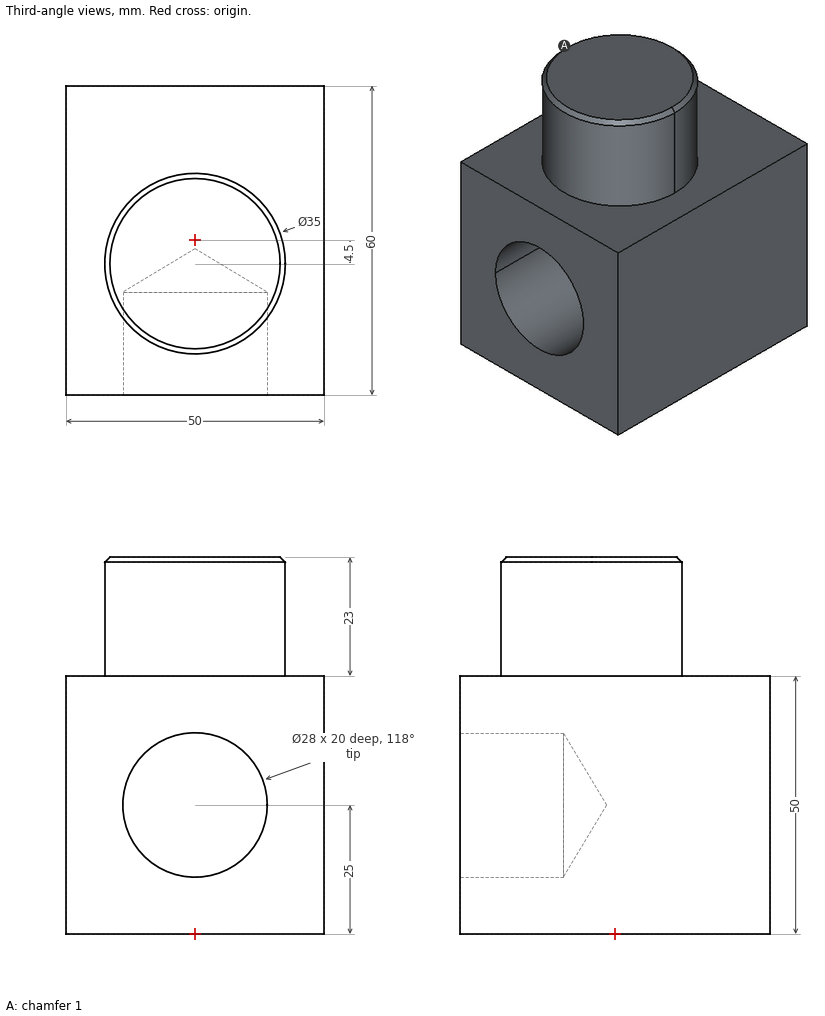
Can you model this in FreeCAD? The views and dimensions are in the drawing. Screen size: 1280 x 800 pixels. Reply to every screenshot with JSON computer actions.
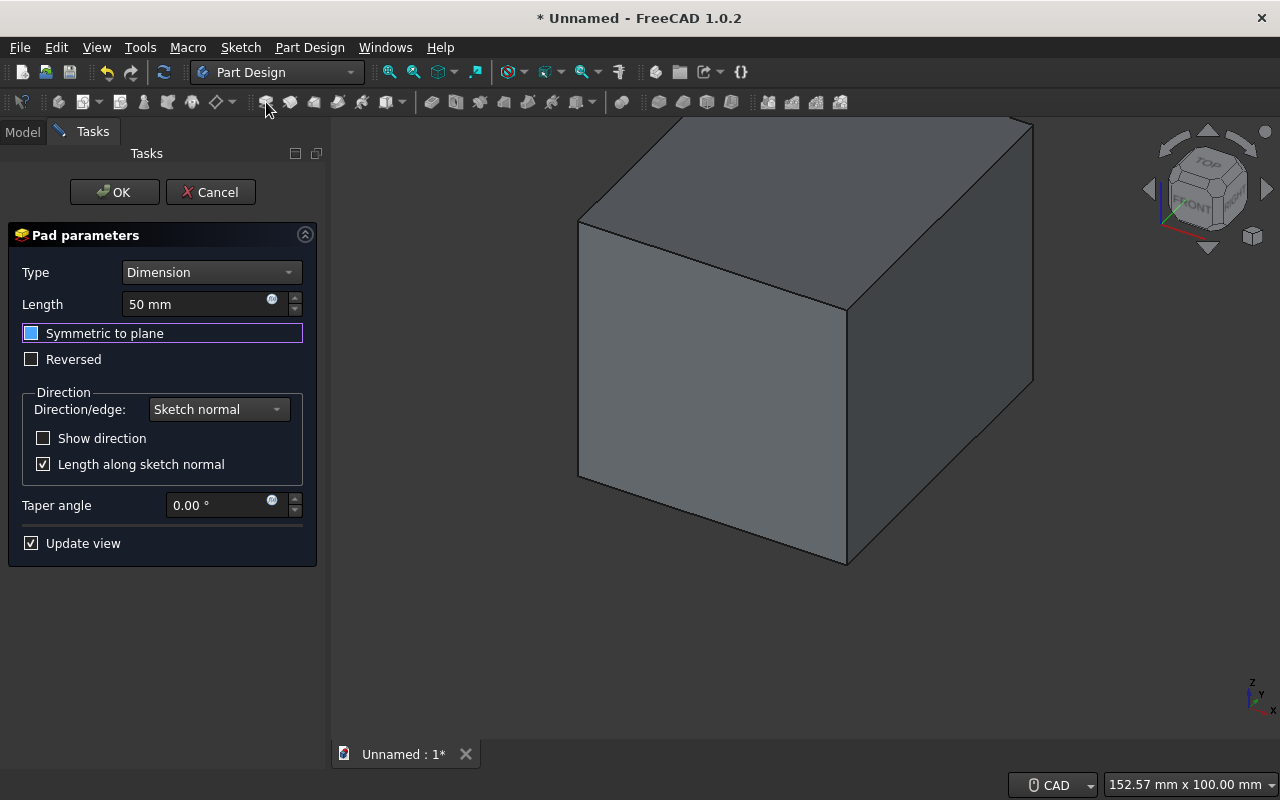
{"action": "left_click", "coordinate": [115, 192]}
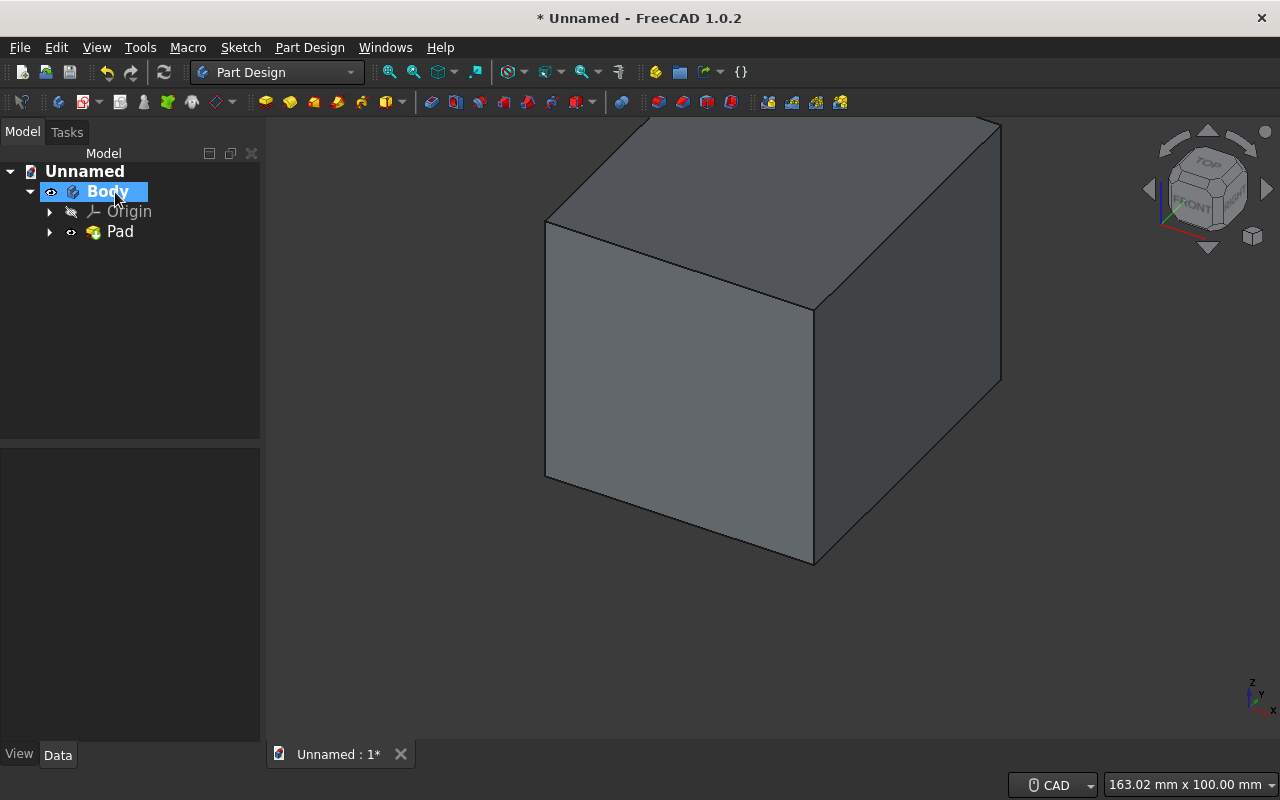
{"action": "left_click", "coordinate": [390, 72]}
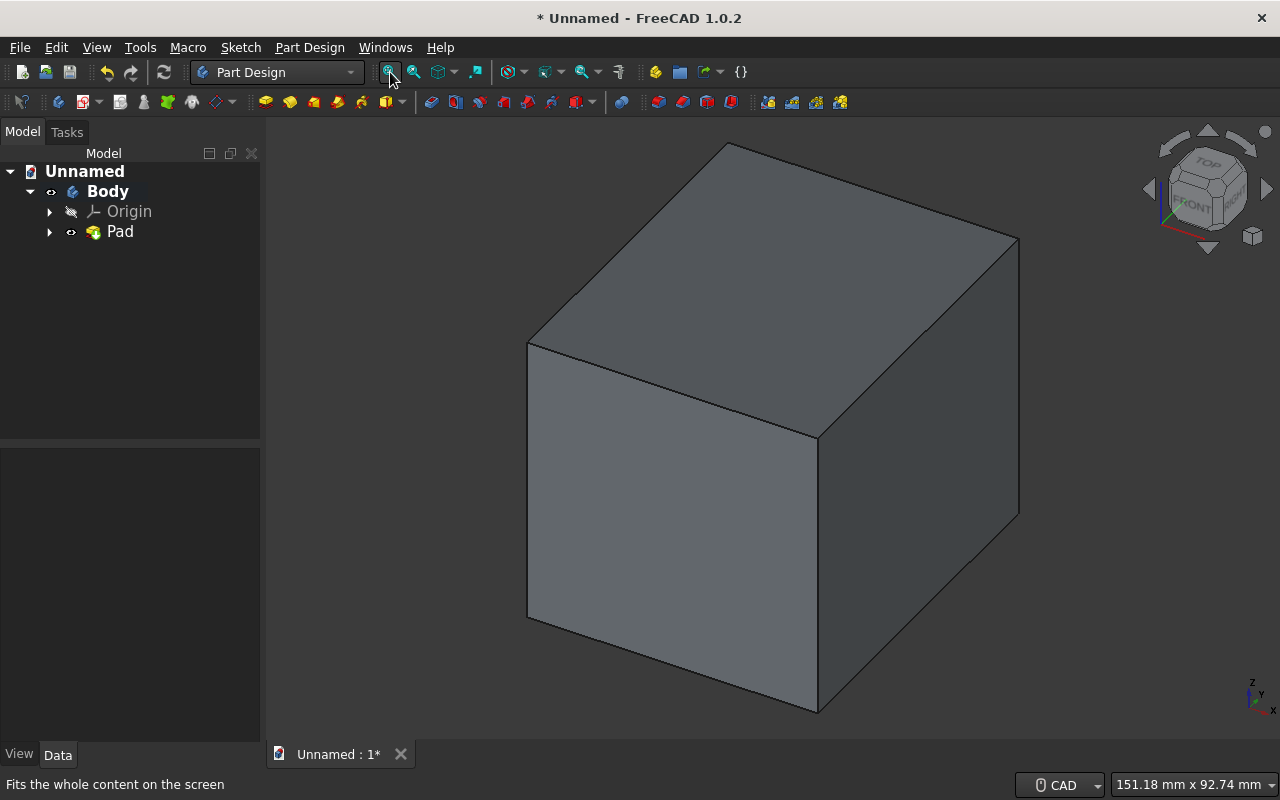
{"action": "left_click", "coordinate": [773, 290]}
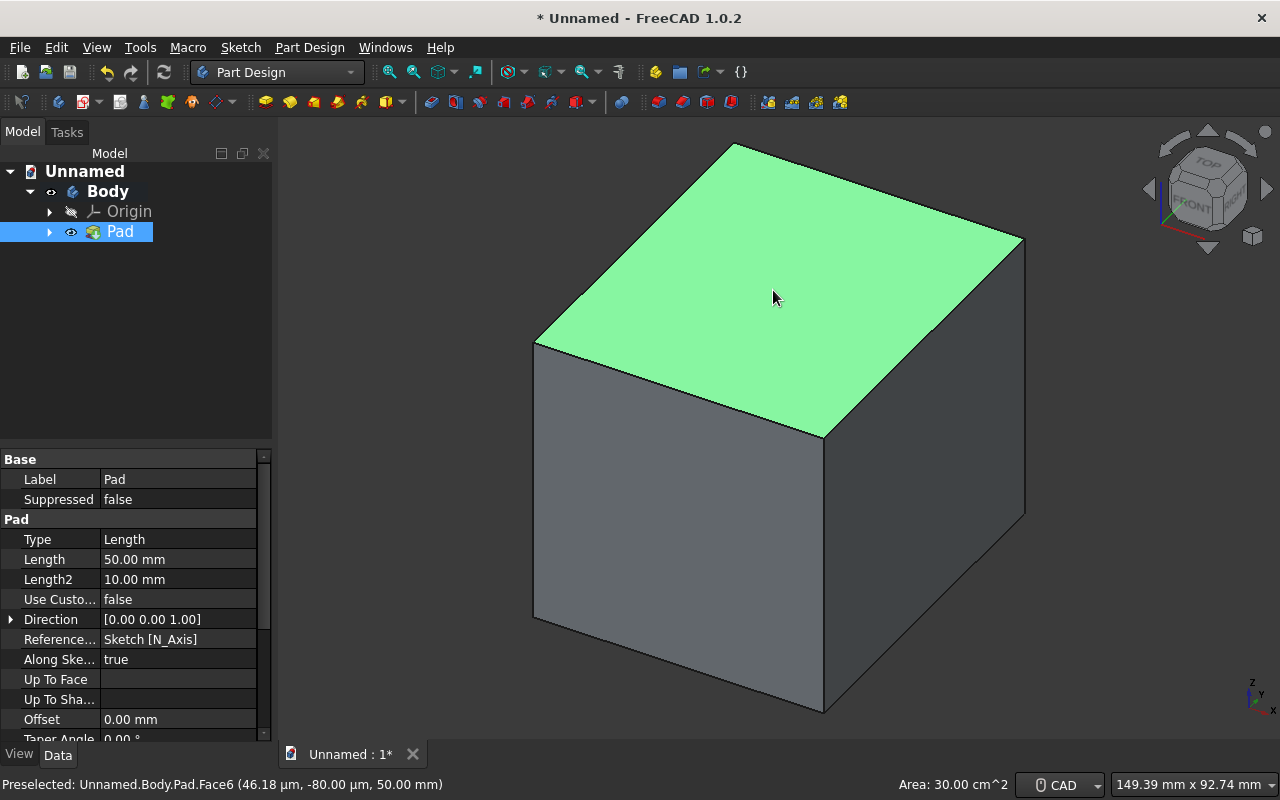
{"action": "left_click", "coordinate": [84, 102]}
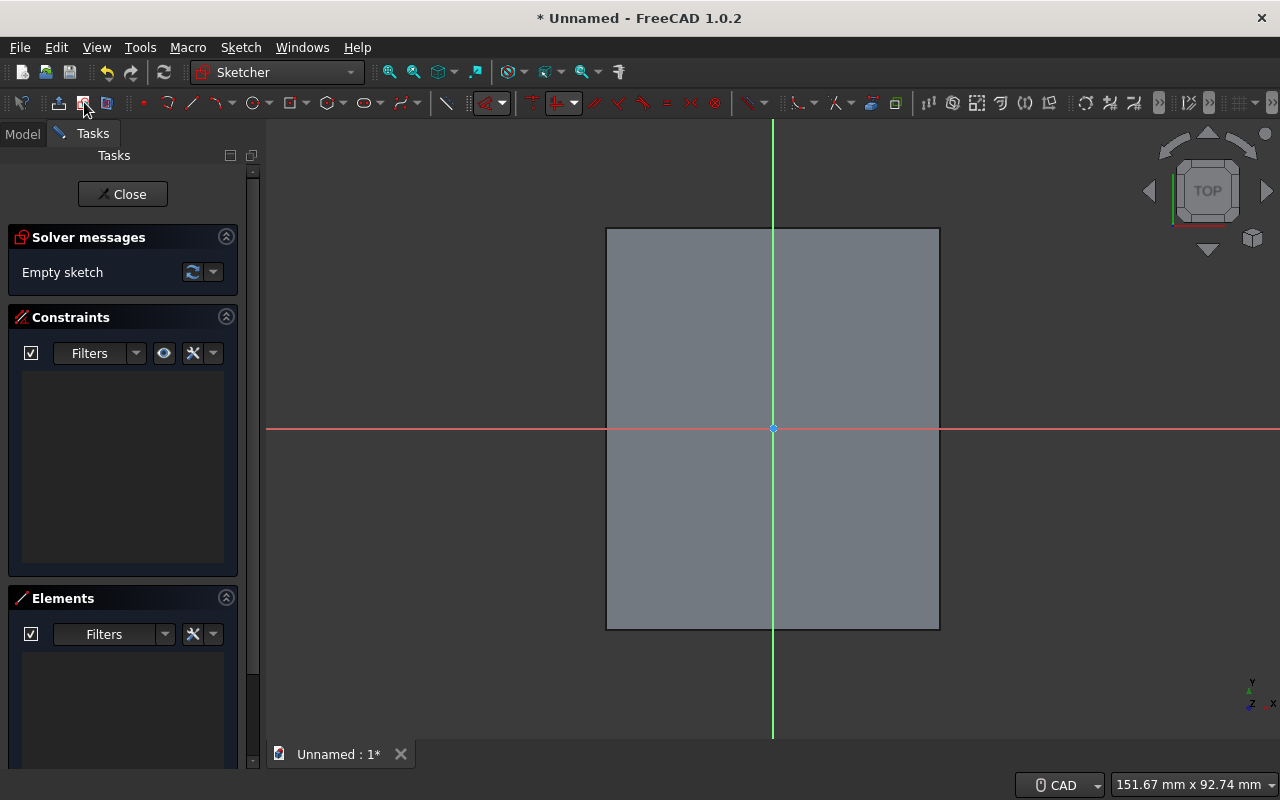
{"action": "scroll", "coordinate": [856, 496], "scroll_direction": "up", "scroll_amount": 3}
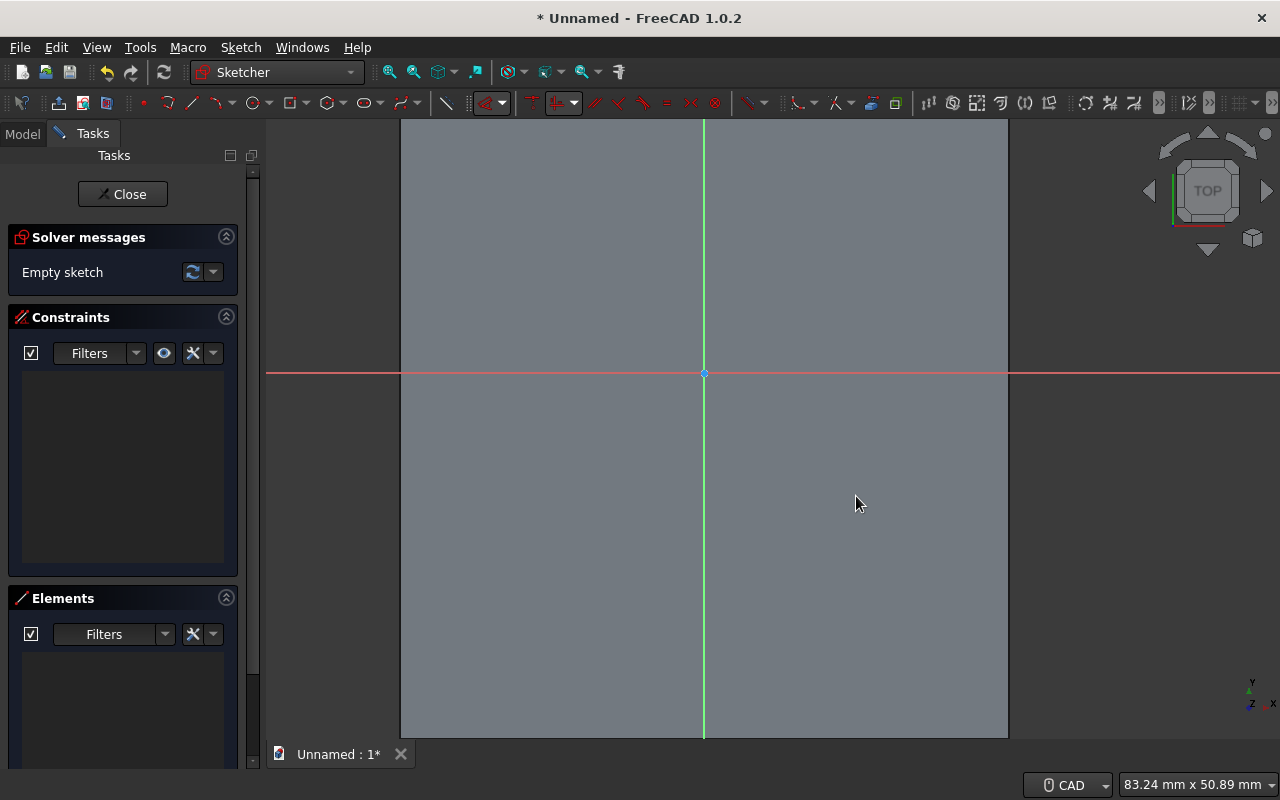
{"action": "left_click", "coordinate": [254, 104]}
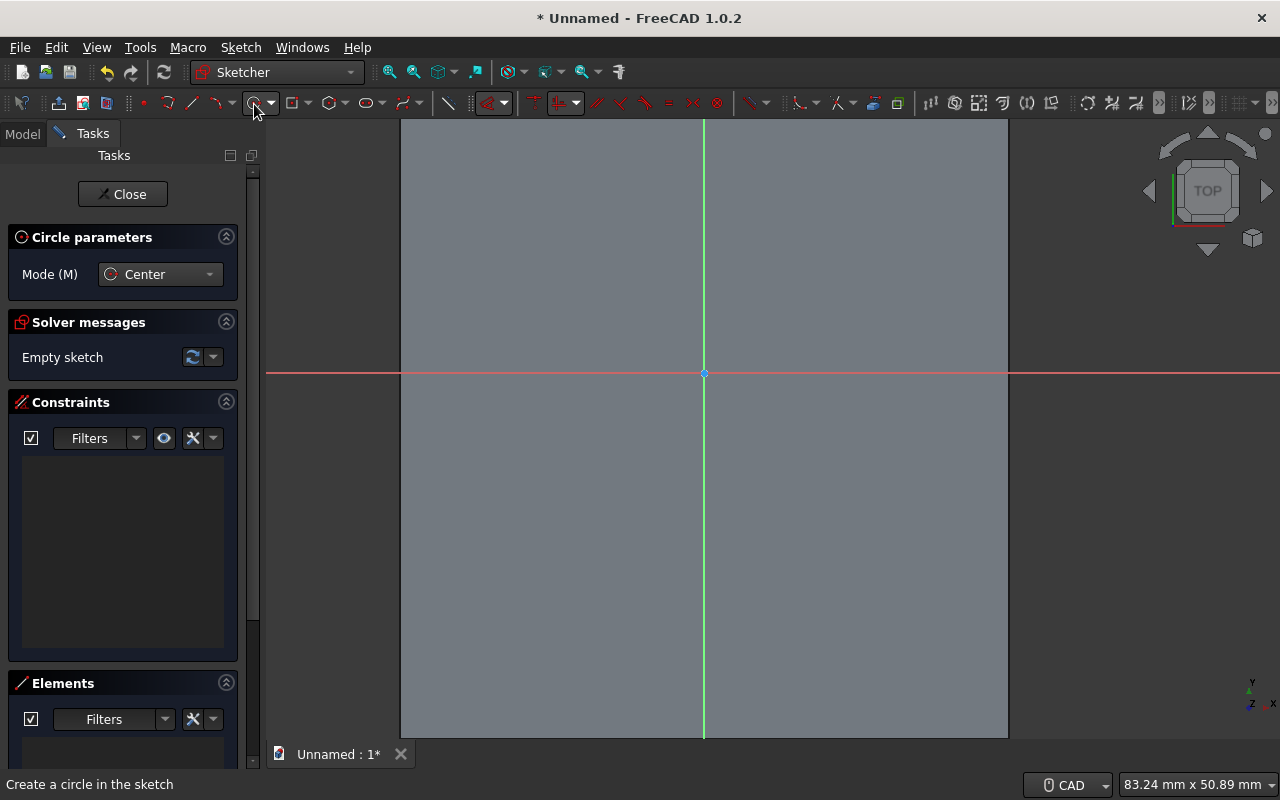
{"action": "left_click", "coordinate": [704, 428]}
{"action": "mouse_move", "coordinate": [855, 277]}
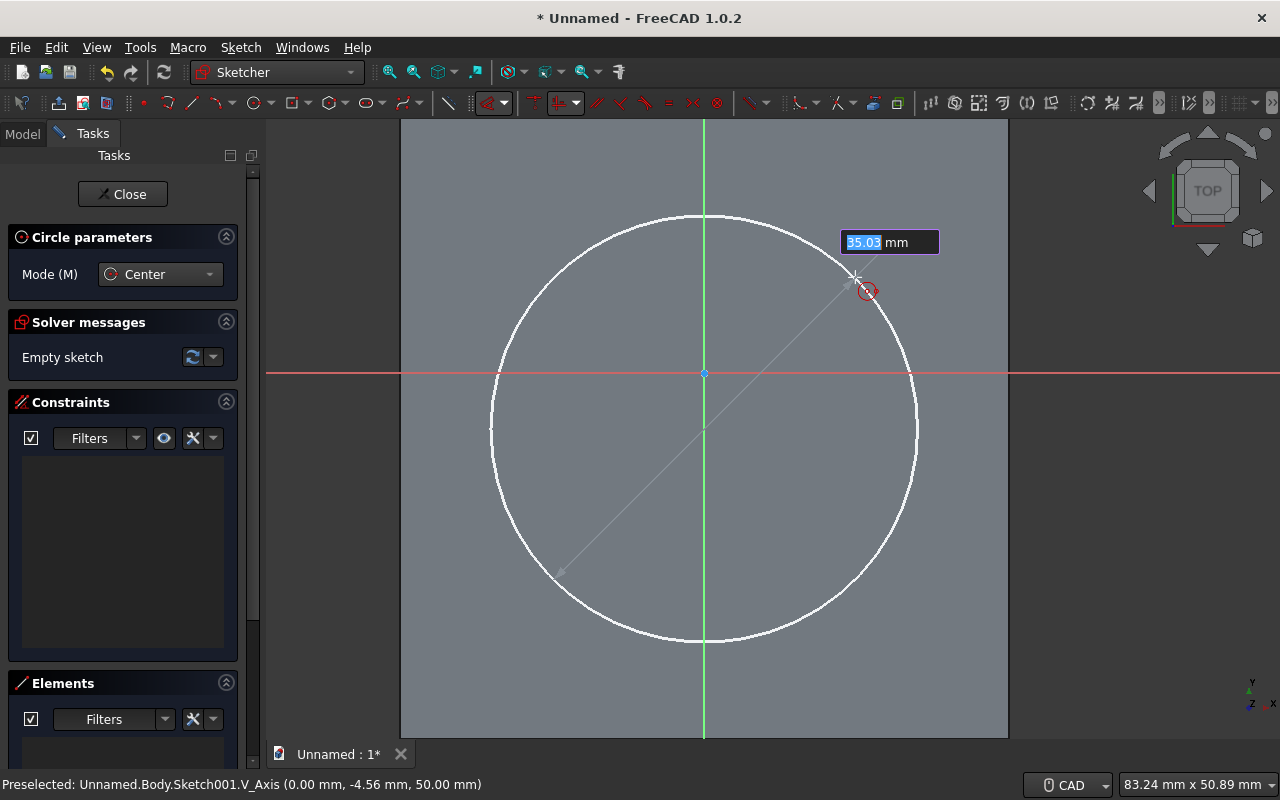
{"action": "type", "text": "35"}
{"action": "key", "text": "Return"}
{"action": "key", "text": "Escape"}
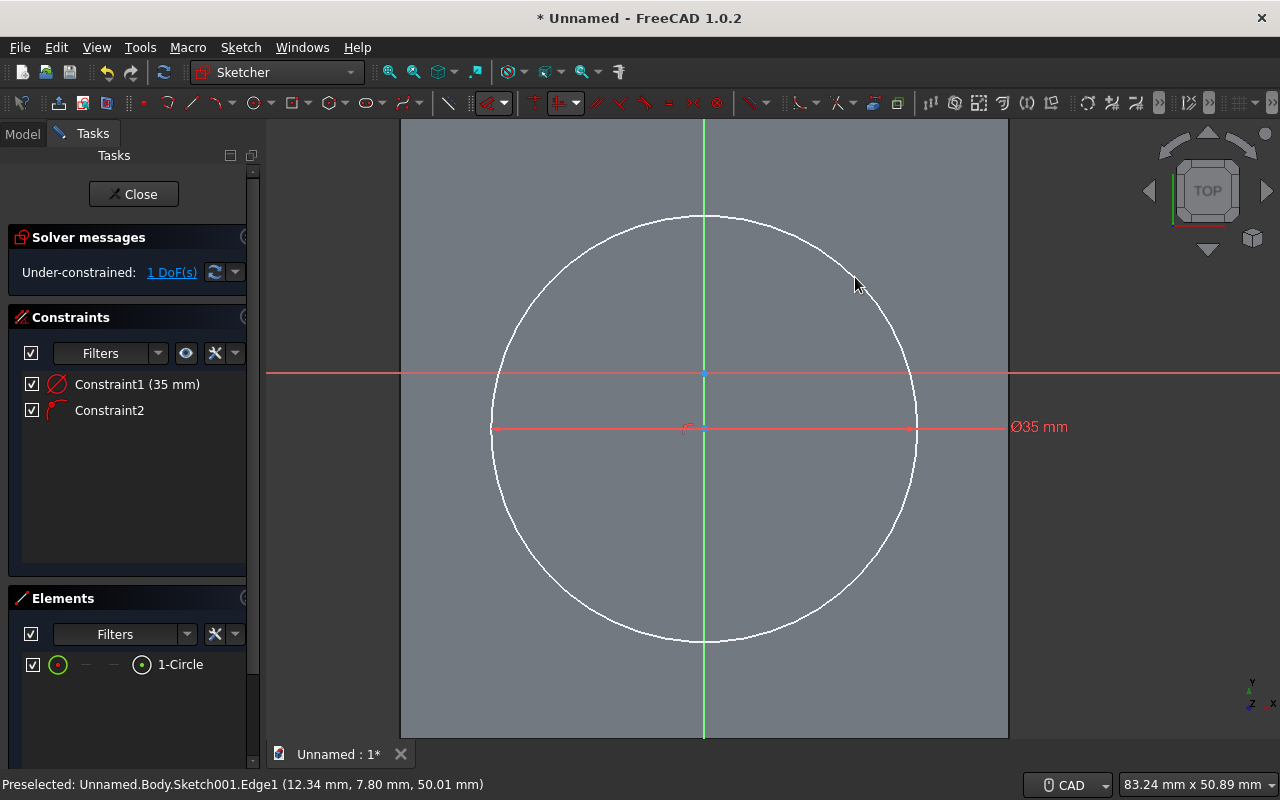
{"action": "left_click", "coordinate": [488, 104]}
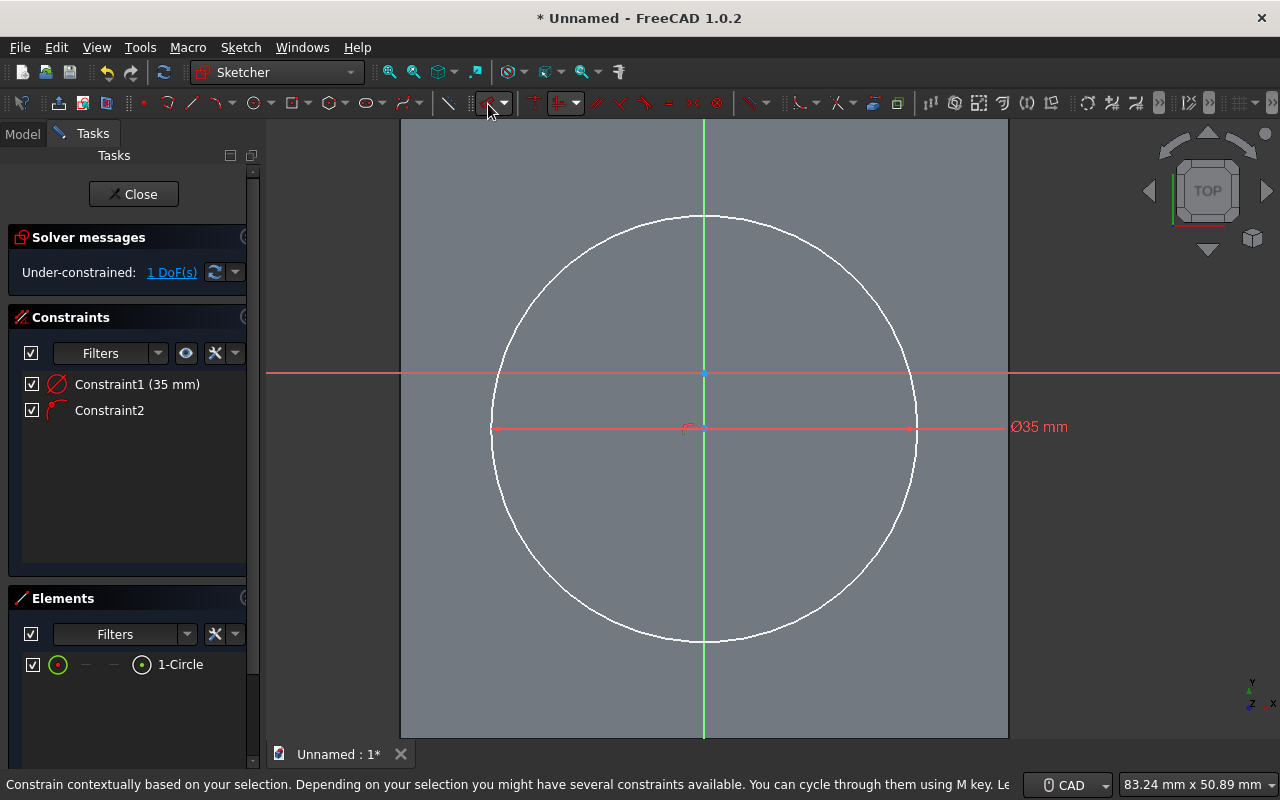
{"action": "left_click", "coordinate": [704, 429]}
{"action": "left_click", "coordinate": [738, 401]}